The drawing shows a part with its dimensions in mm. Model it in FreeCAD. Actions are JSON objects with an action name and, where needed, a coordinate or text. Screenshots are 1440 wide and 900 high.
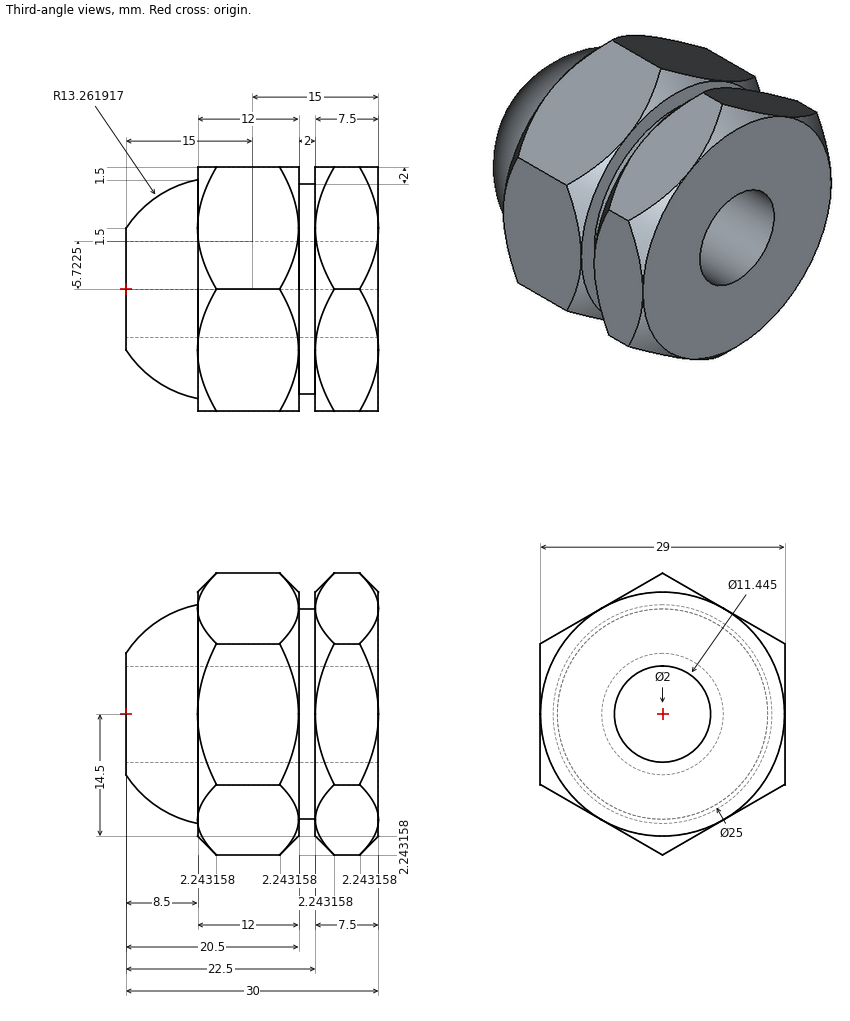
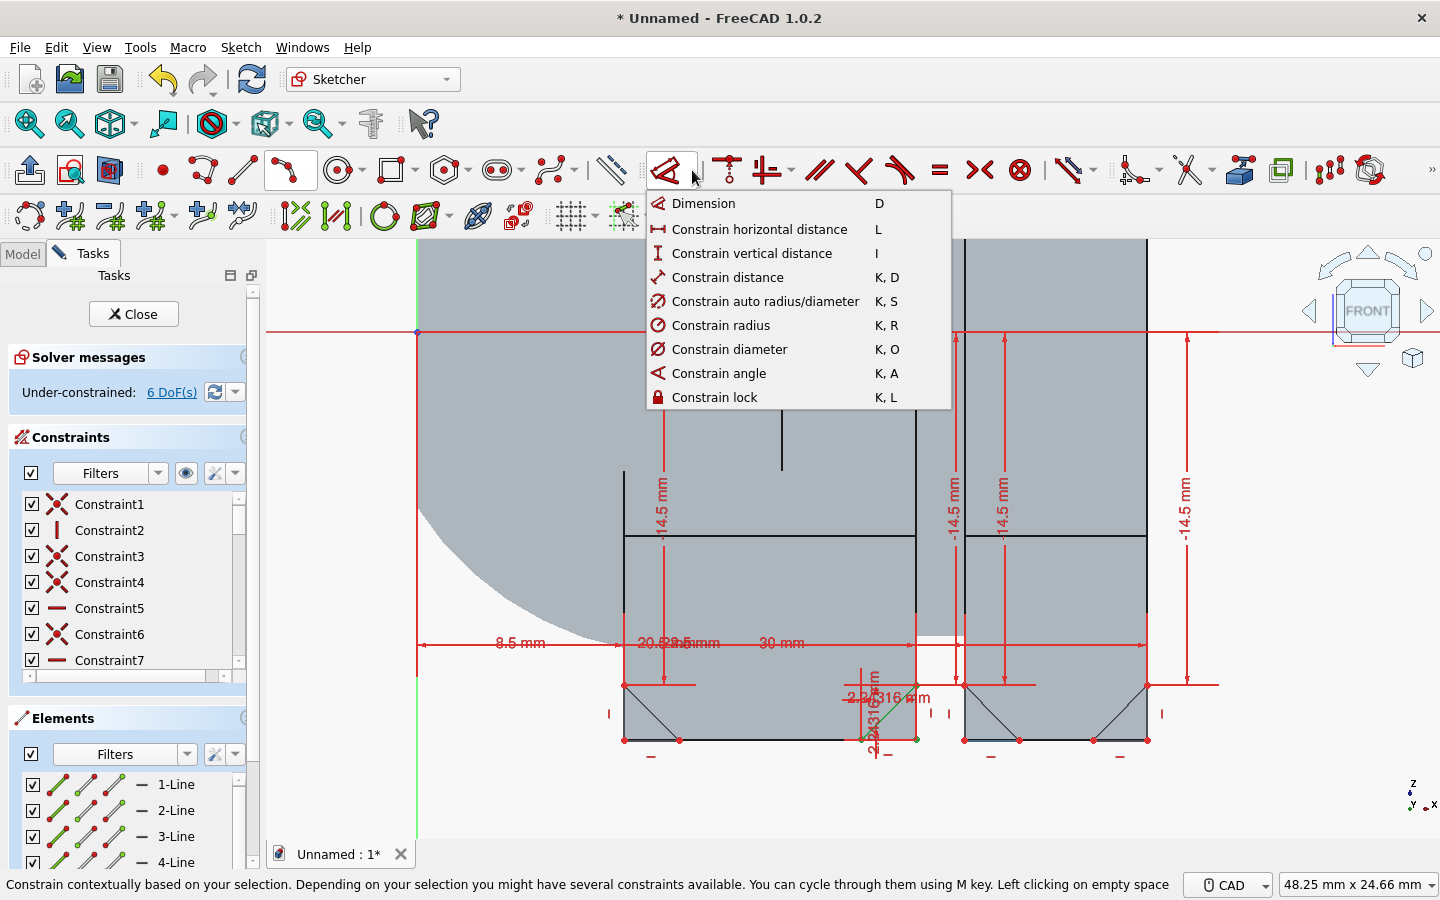
{"action": "left_click", "coordinate": [799, 229]}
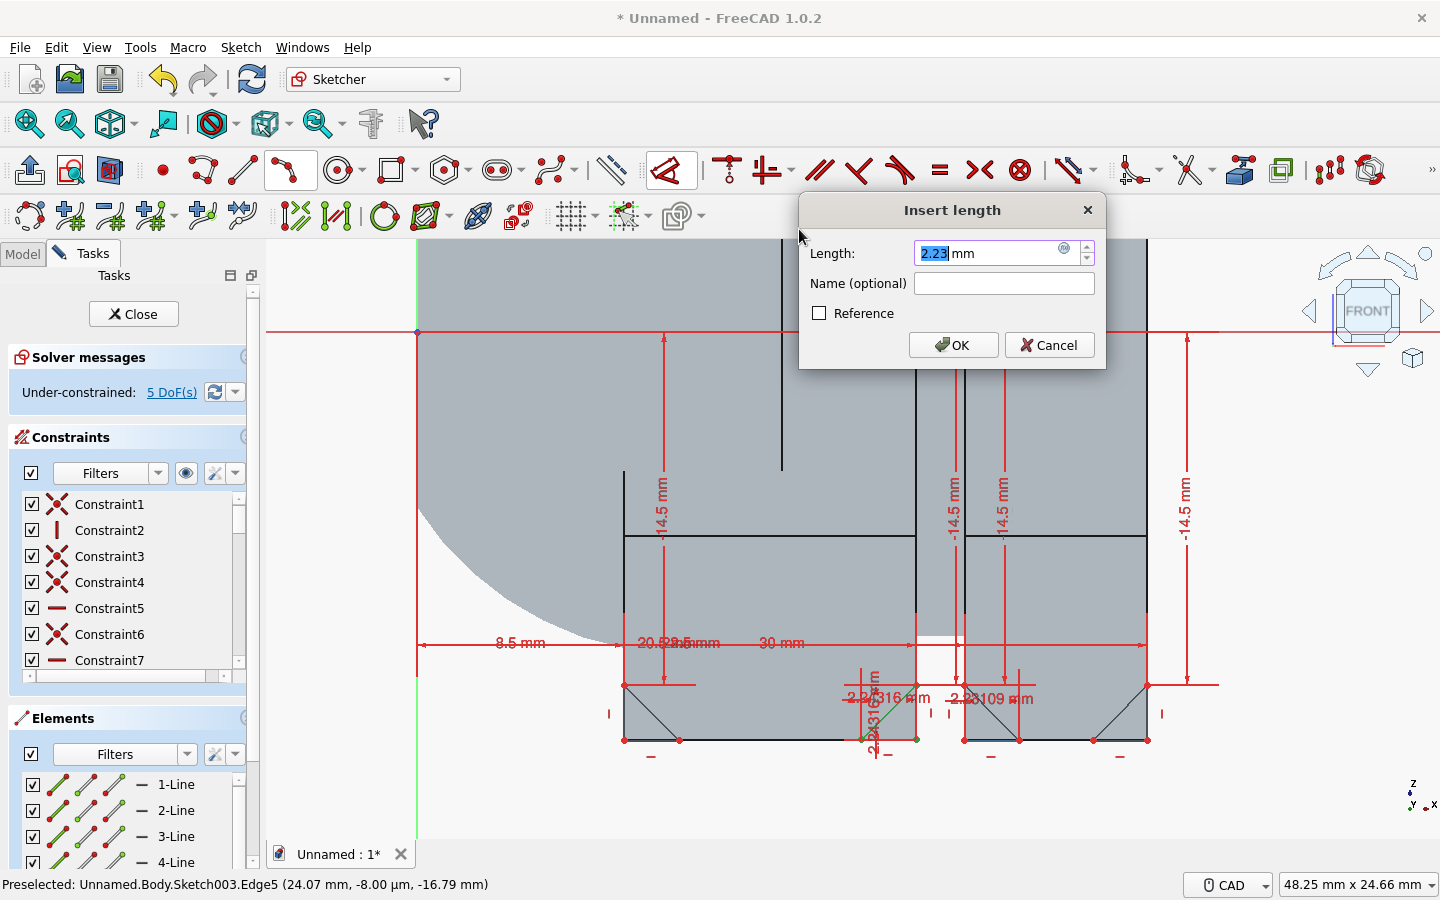
{"action": "type", "text": "2.243158"}
{"action": "key", "text": "Return"}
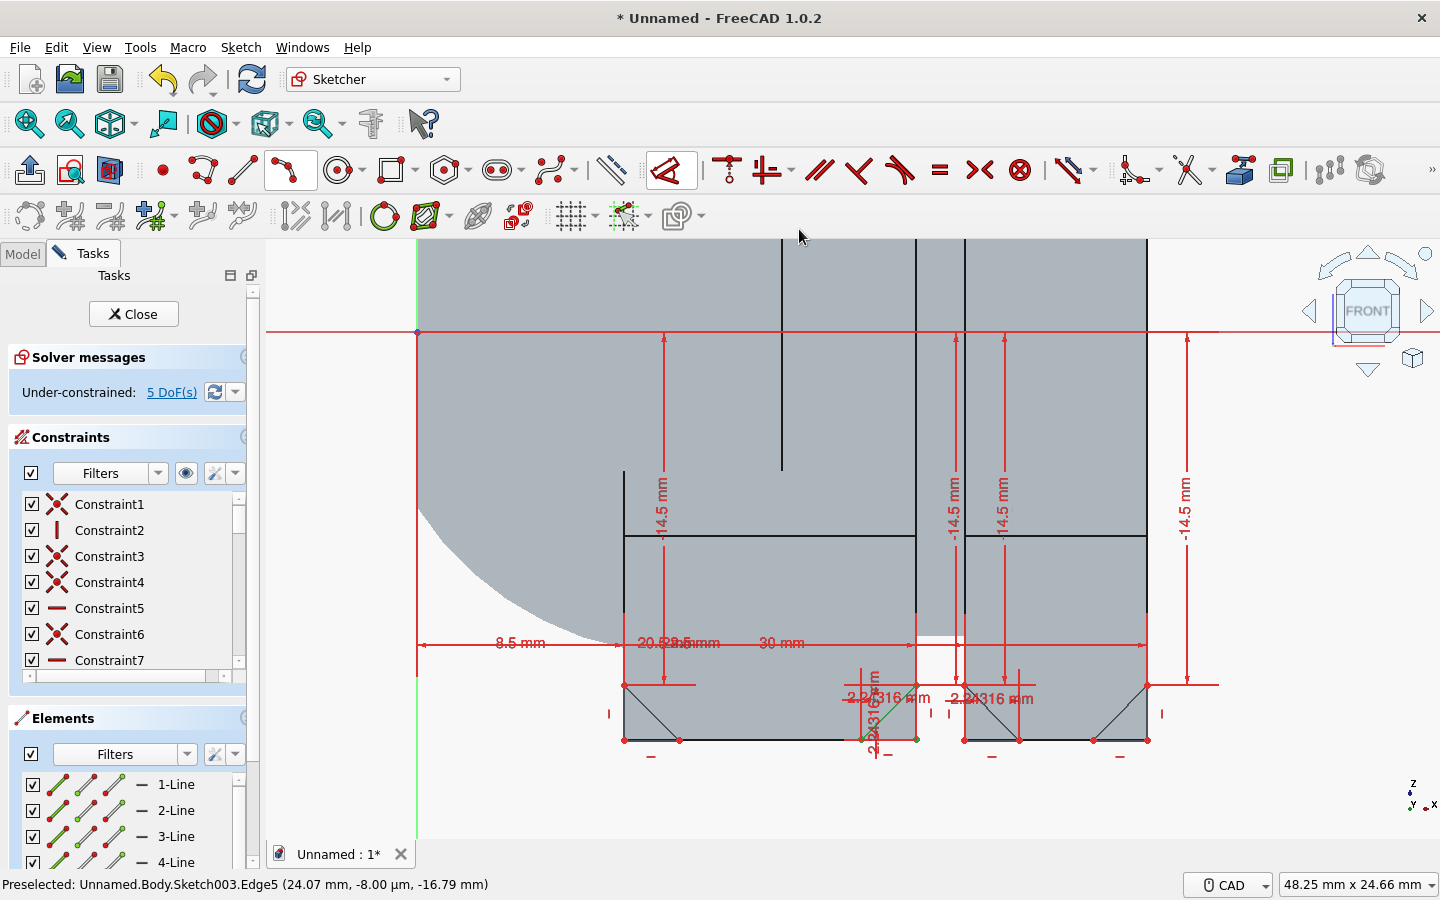
{"action": "left_click", "coordinate": [965, 724]}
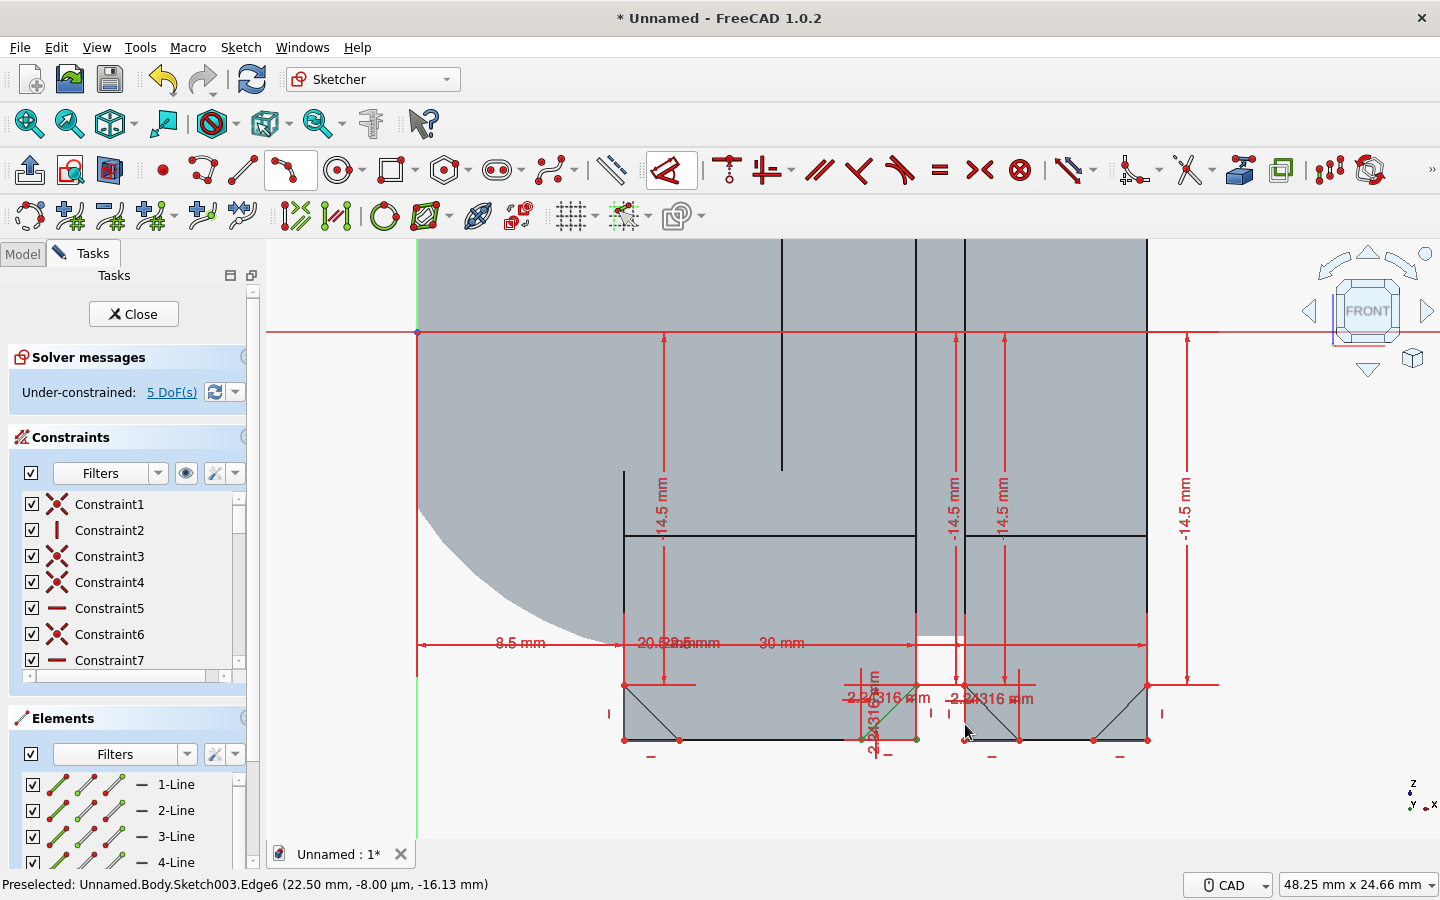
{"action": "left_click", "coordinate": [692, 170]}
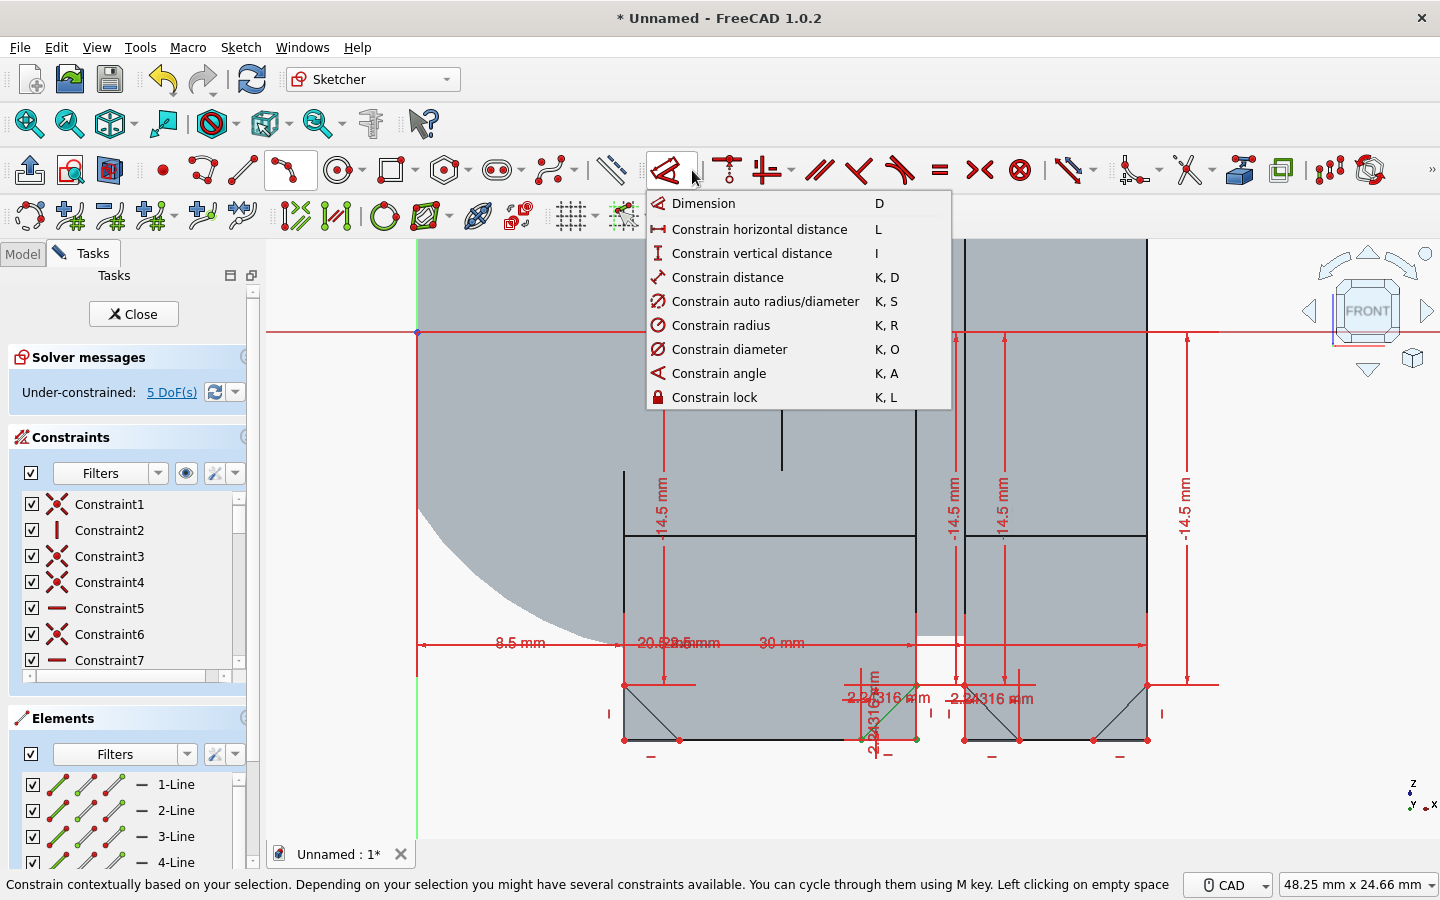
{"action": "left_click", "coordinate": [799, 253]}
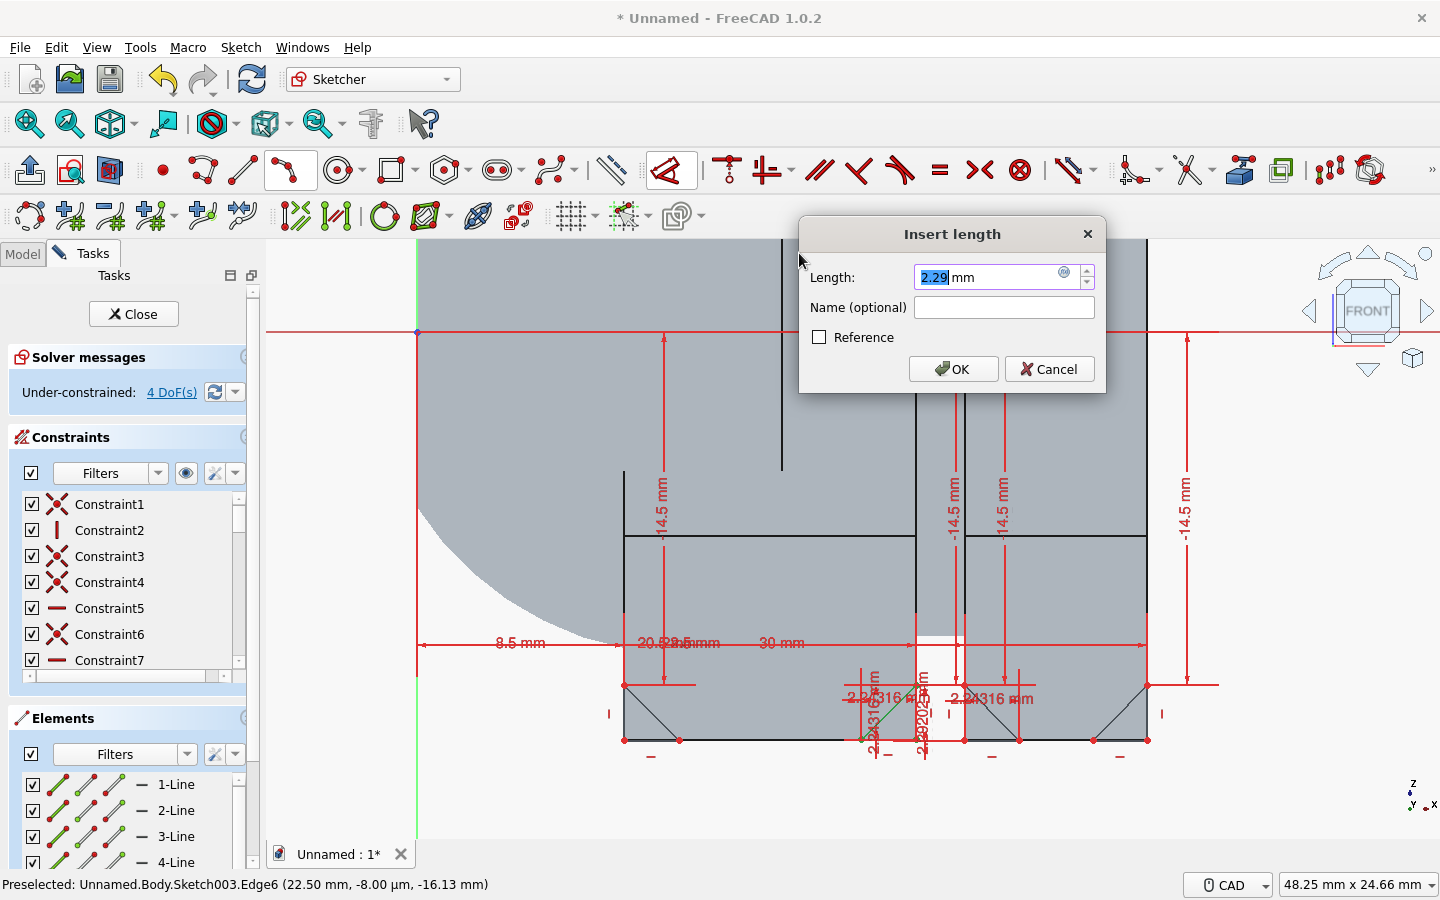
{"action": "type", "text": "2.243158"}
{"action": "key", "text": "Return"}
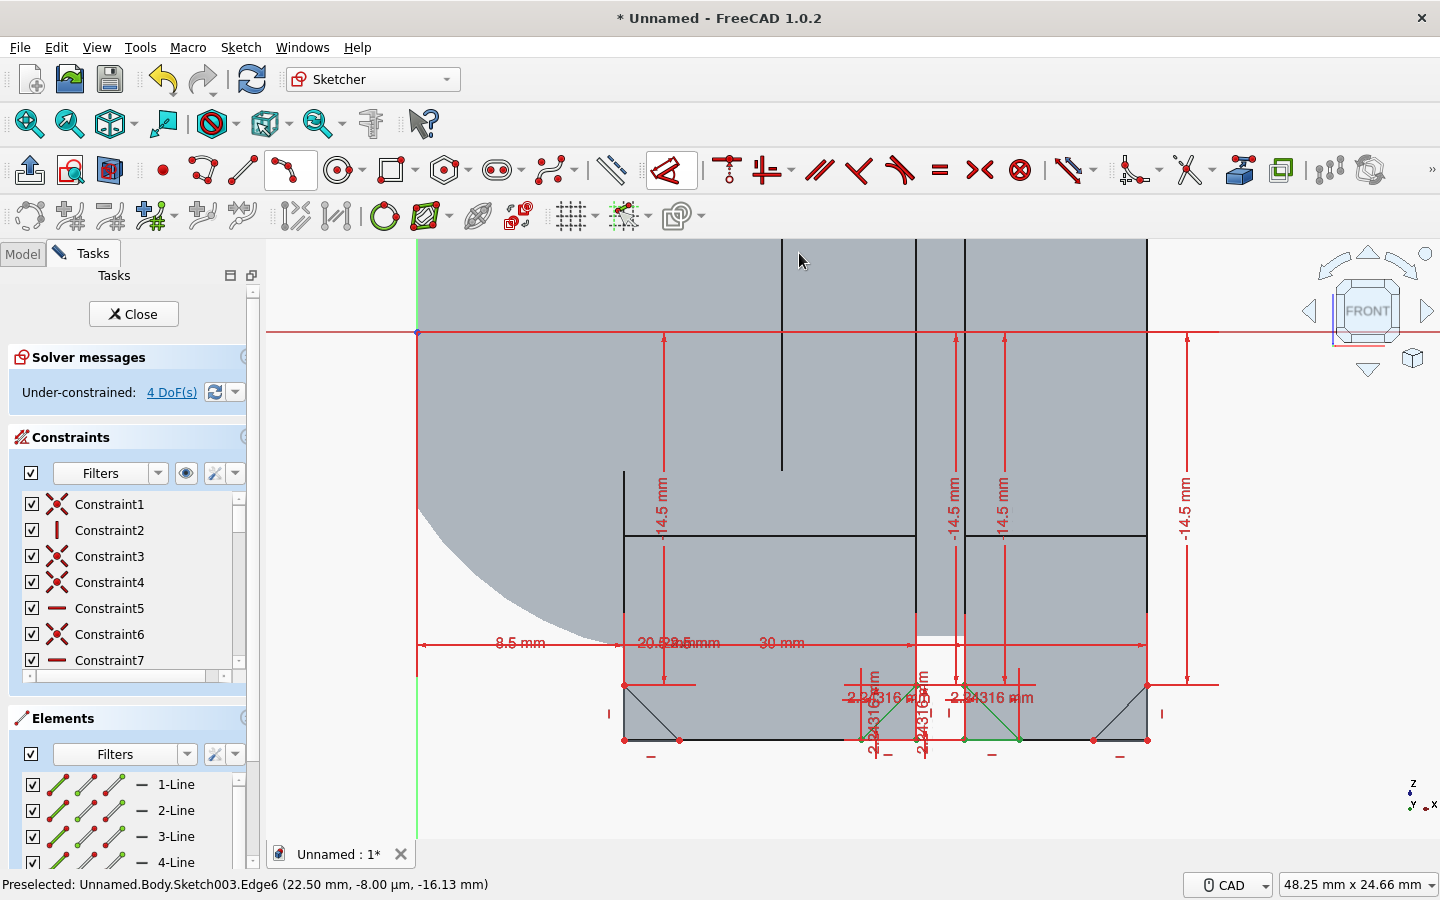
{"action": "left_click", "coordinate": [663, 741]}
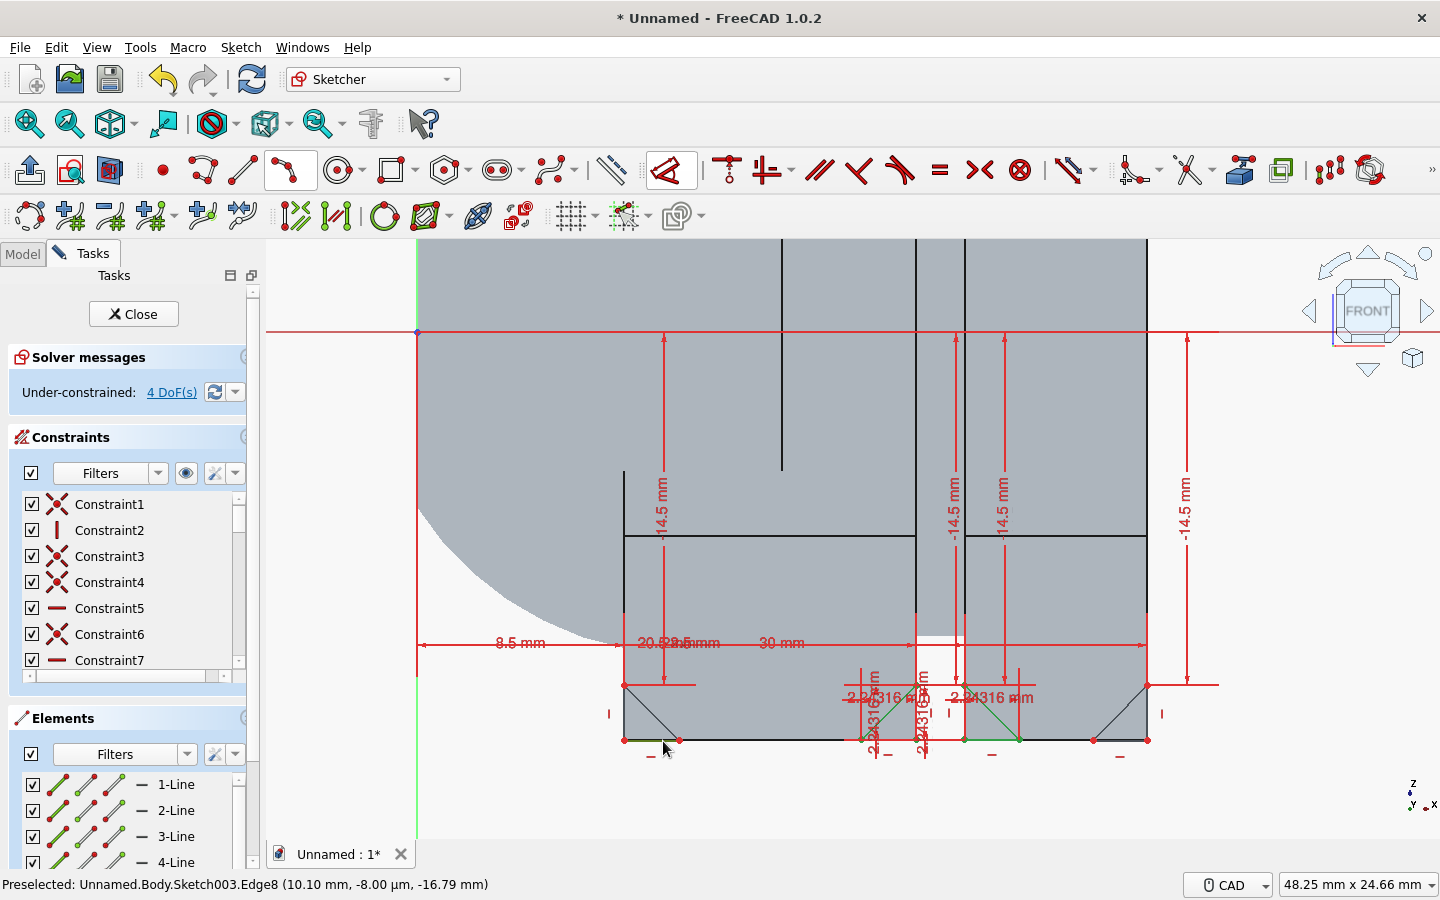
{"action": "left_click", "coordinate": [692, 170]}